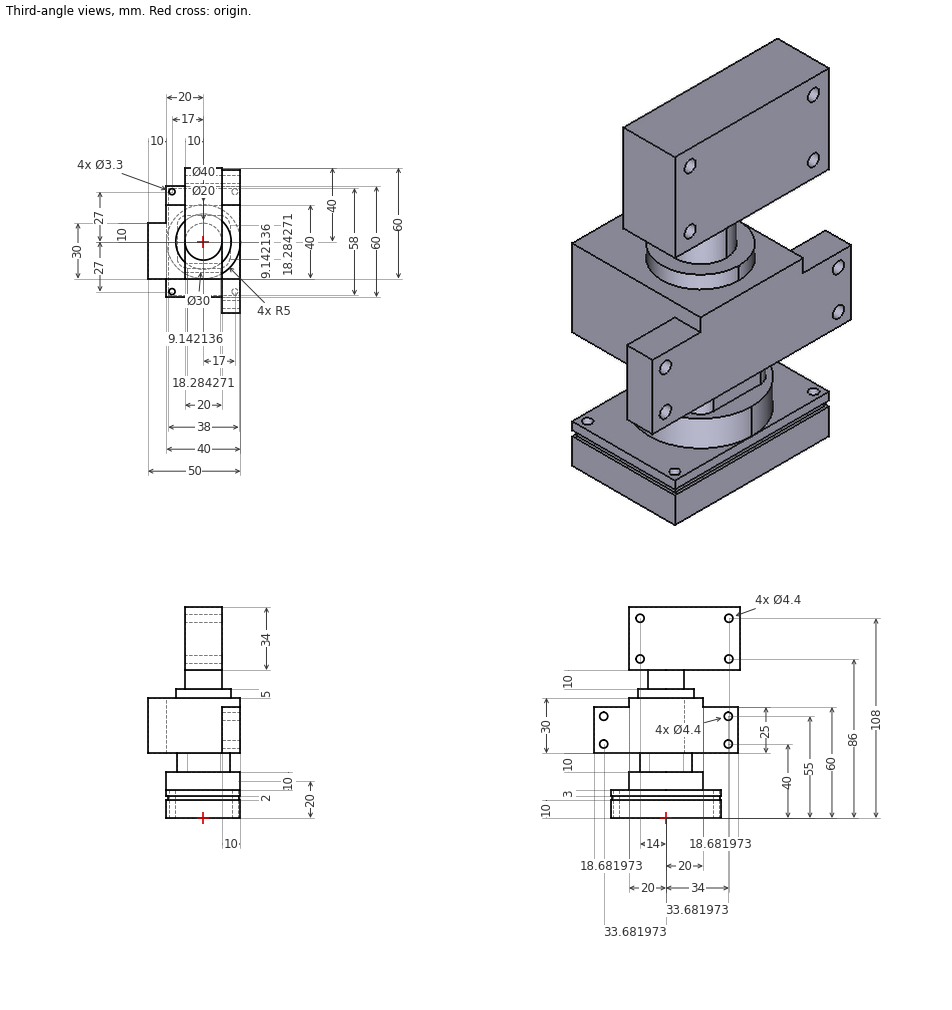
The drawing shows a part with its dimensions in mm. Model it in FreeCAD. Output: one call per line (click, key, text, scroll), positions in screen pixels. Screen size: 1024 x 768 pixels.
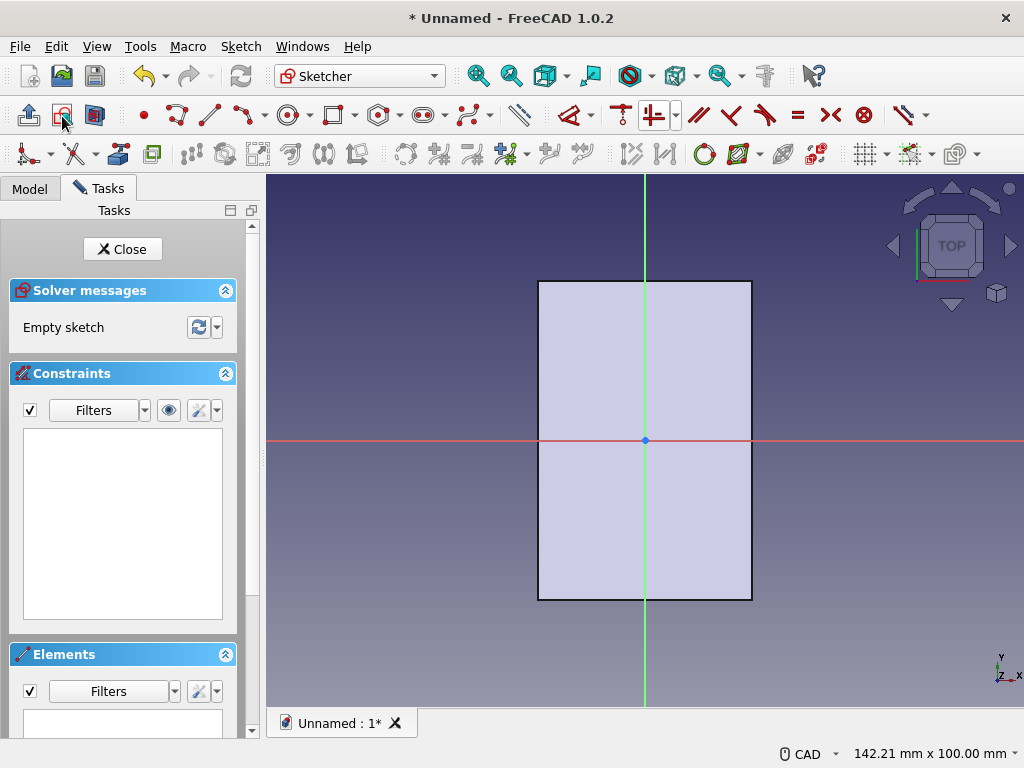
key(g)
key(v)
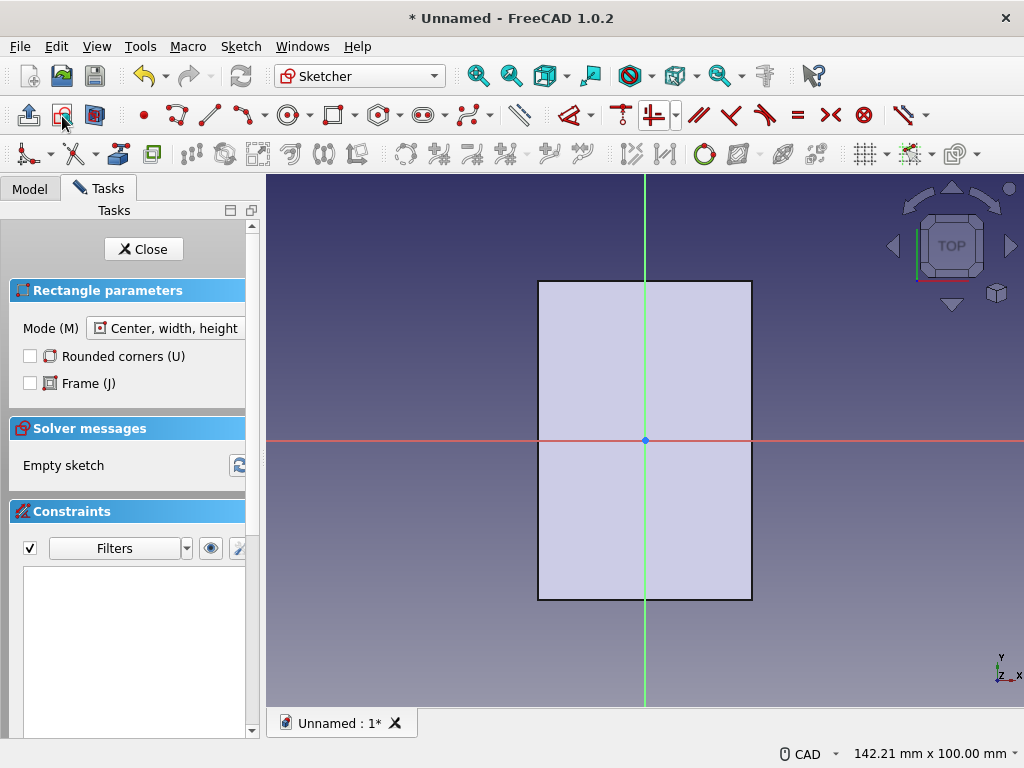
click(645, 440)
move(746, 286)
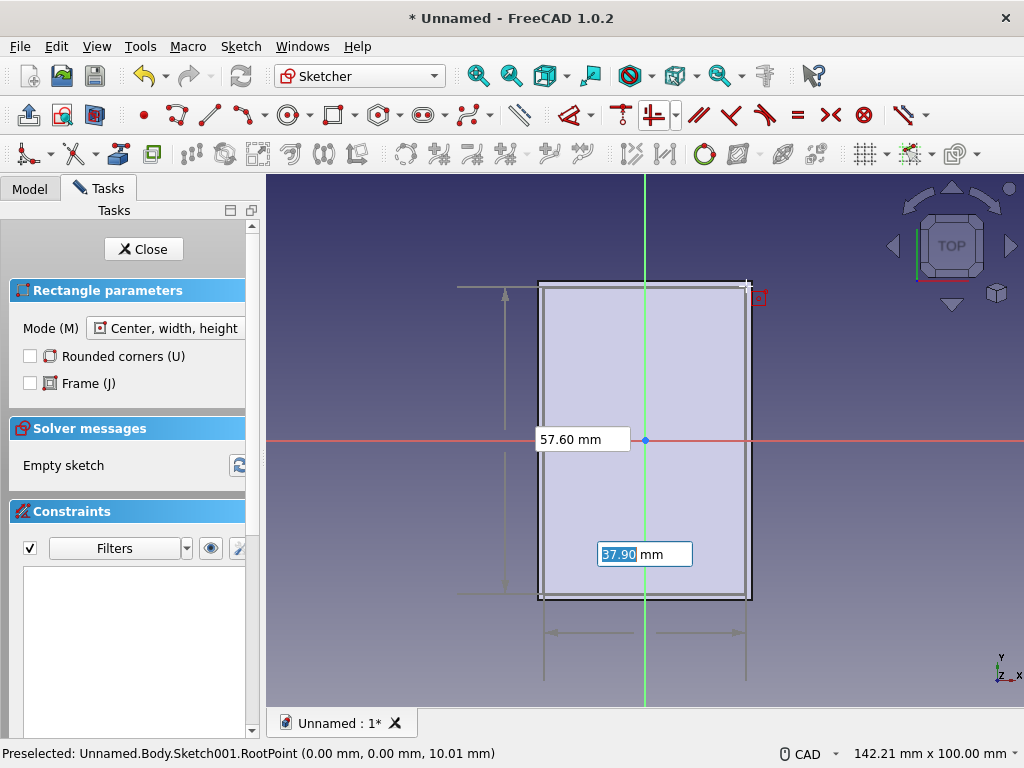
text(38)
key(Tab)
text(58)
key(Return)
key(Escape)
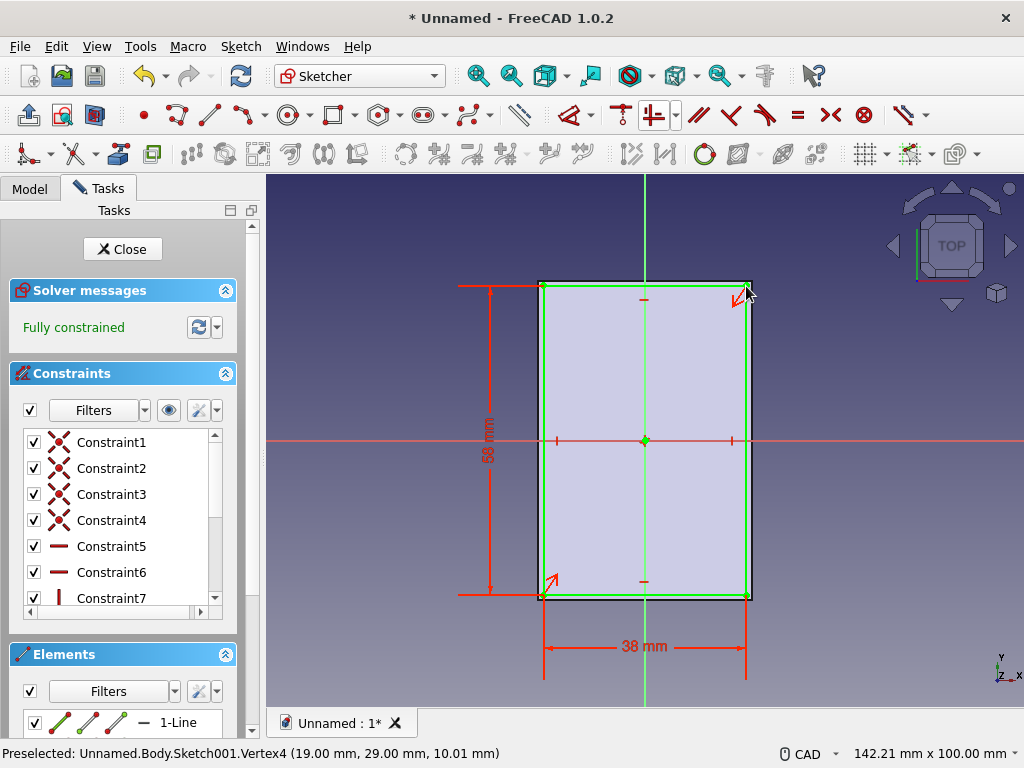
click(123, 249)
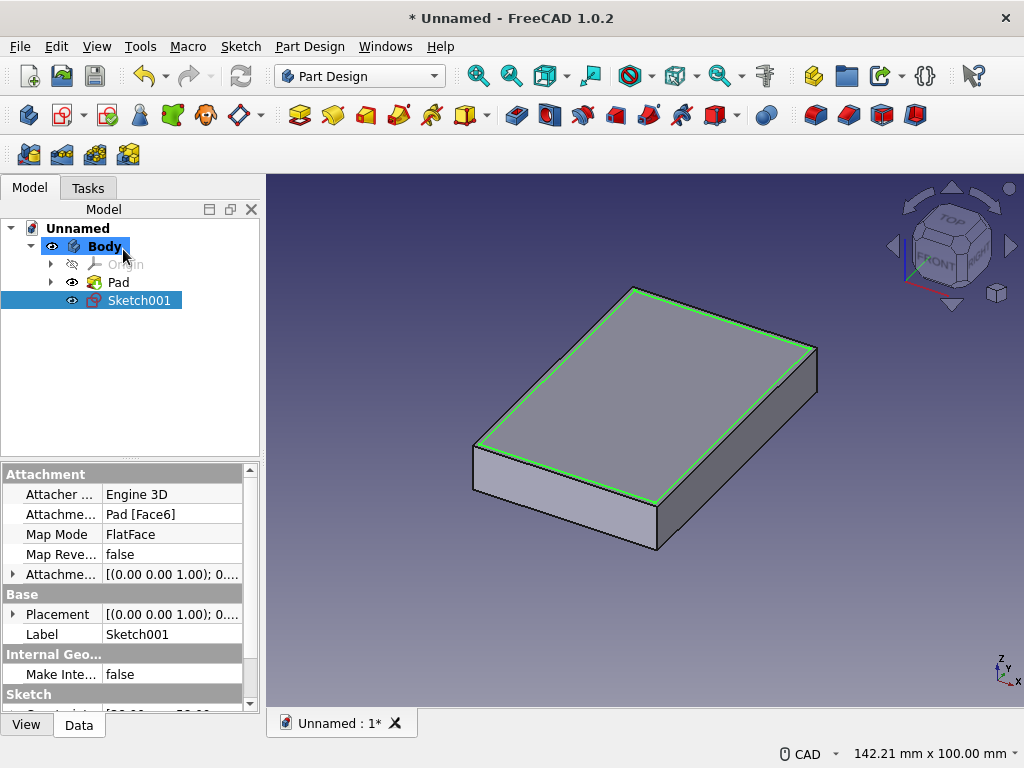
click(300, 116)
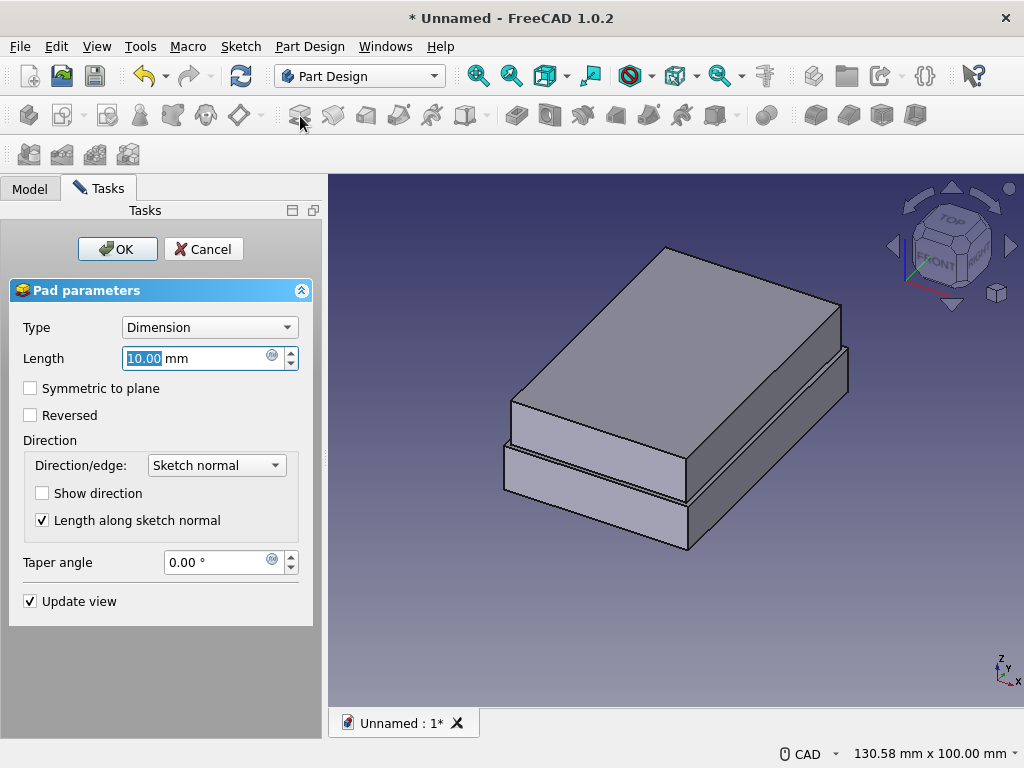
text(2)
key(Tab)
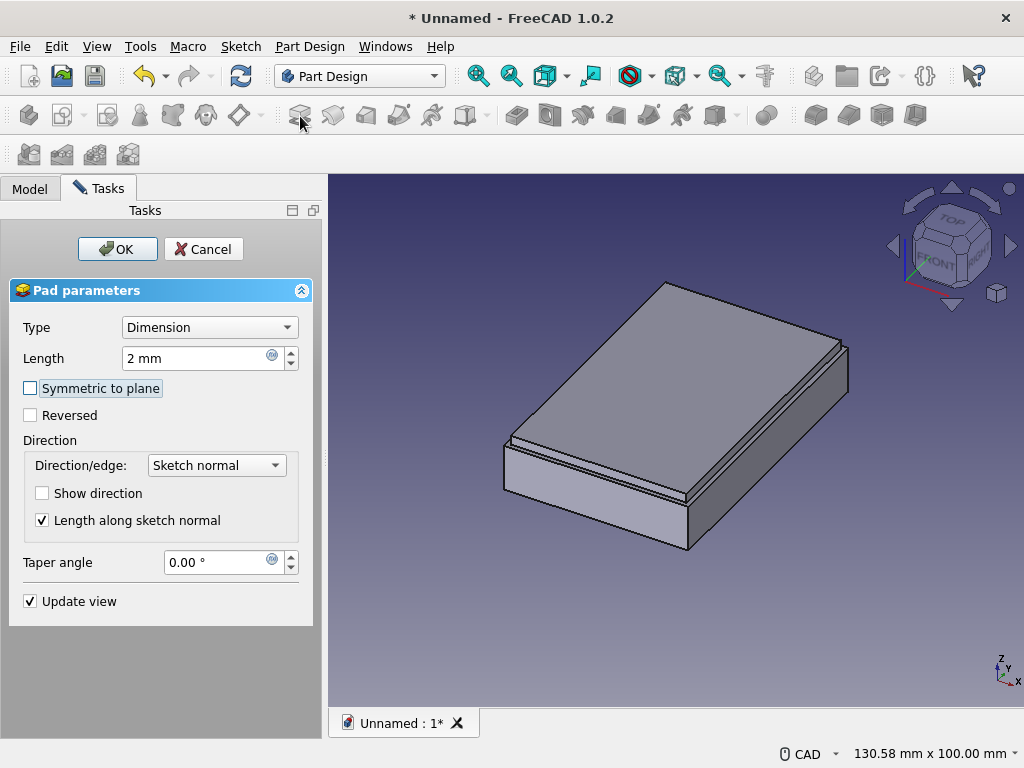
click(118, 249)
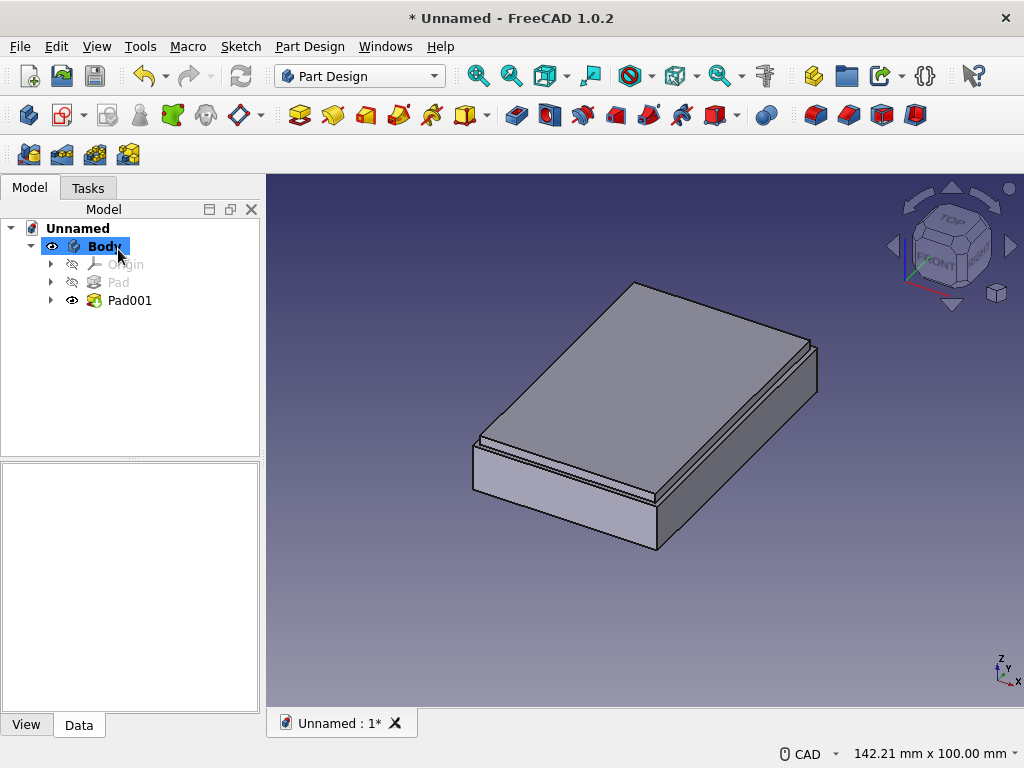
click(667, 365)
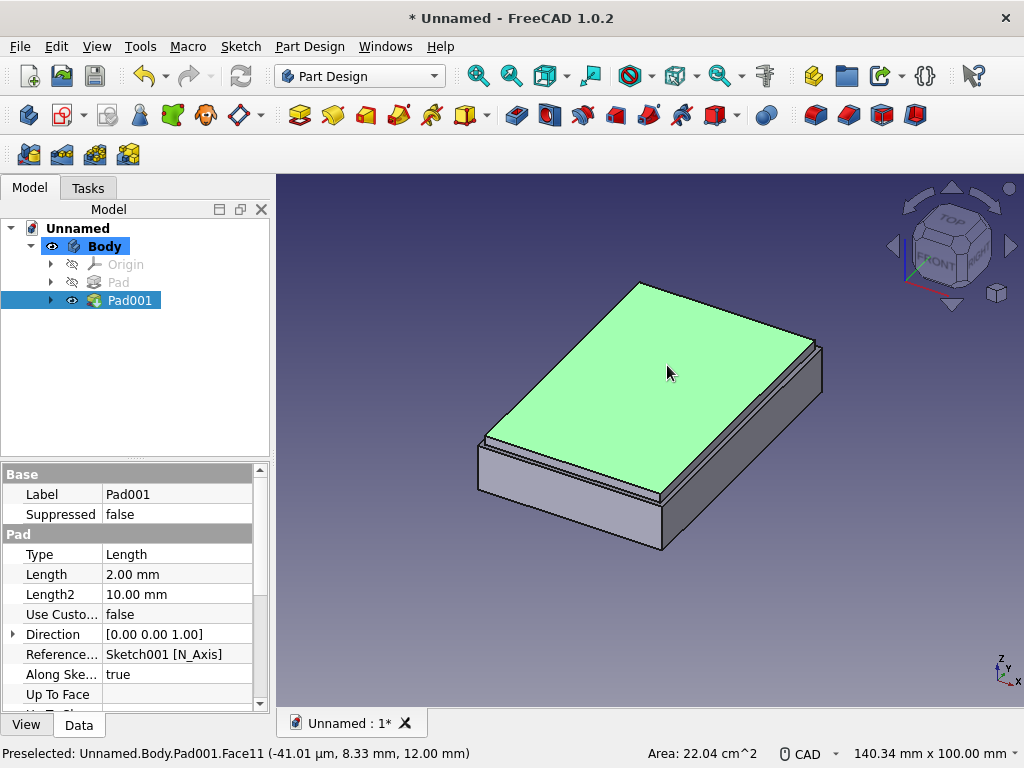
click(62, 116)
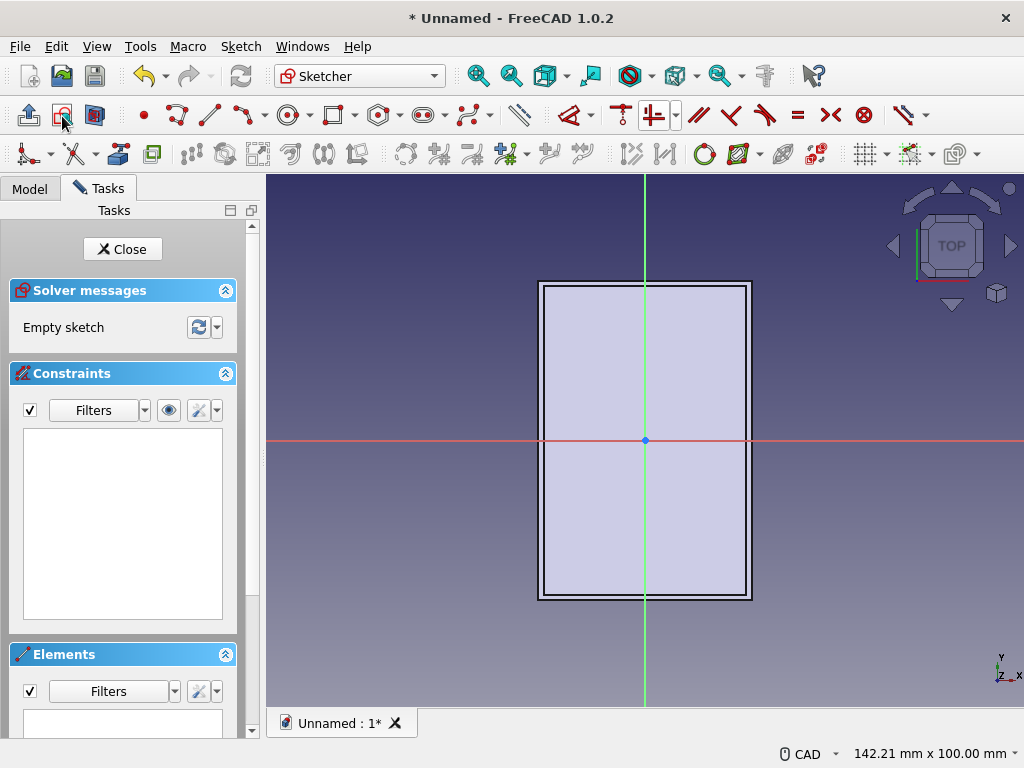
key(g)
key(v)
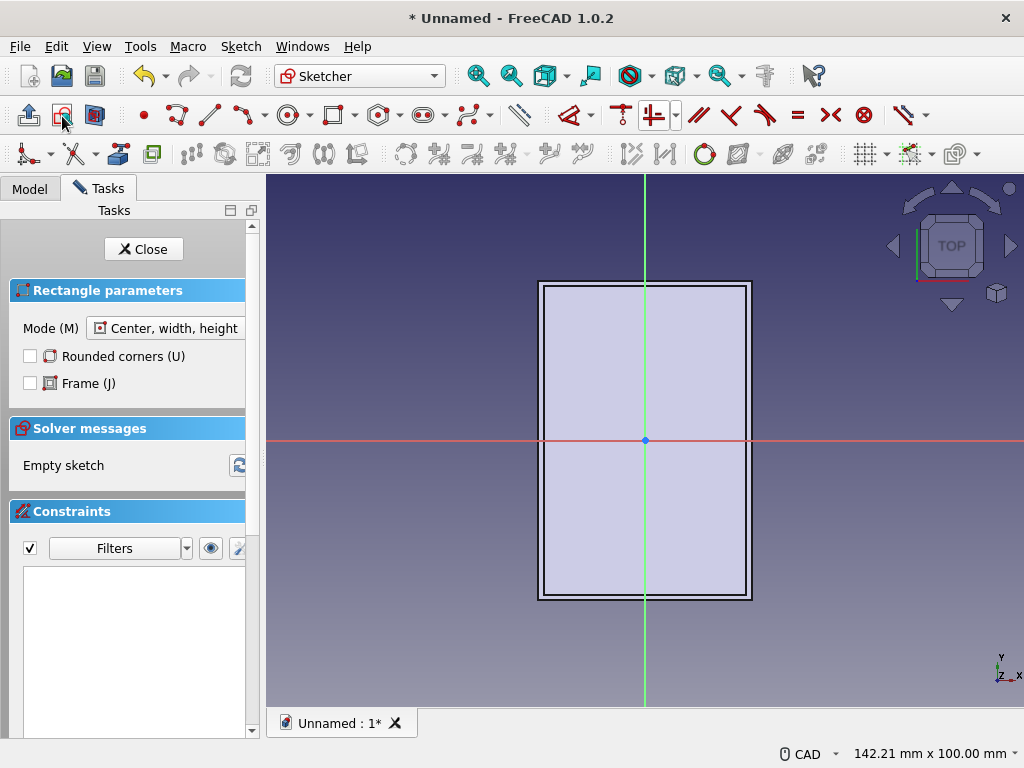
click(645, 440)
move(752, 281)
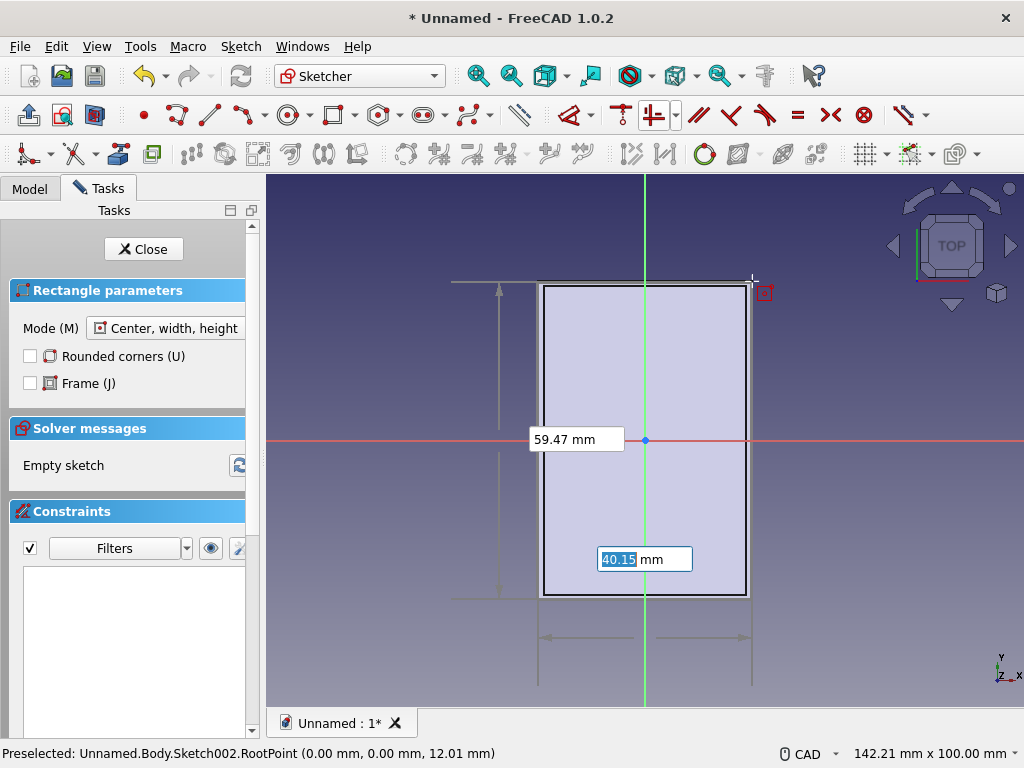
text(40)
key(Tab)
text(60)
key(Return)
key(Escape)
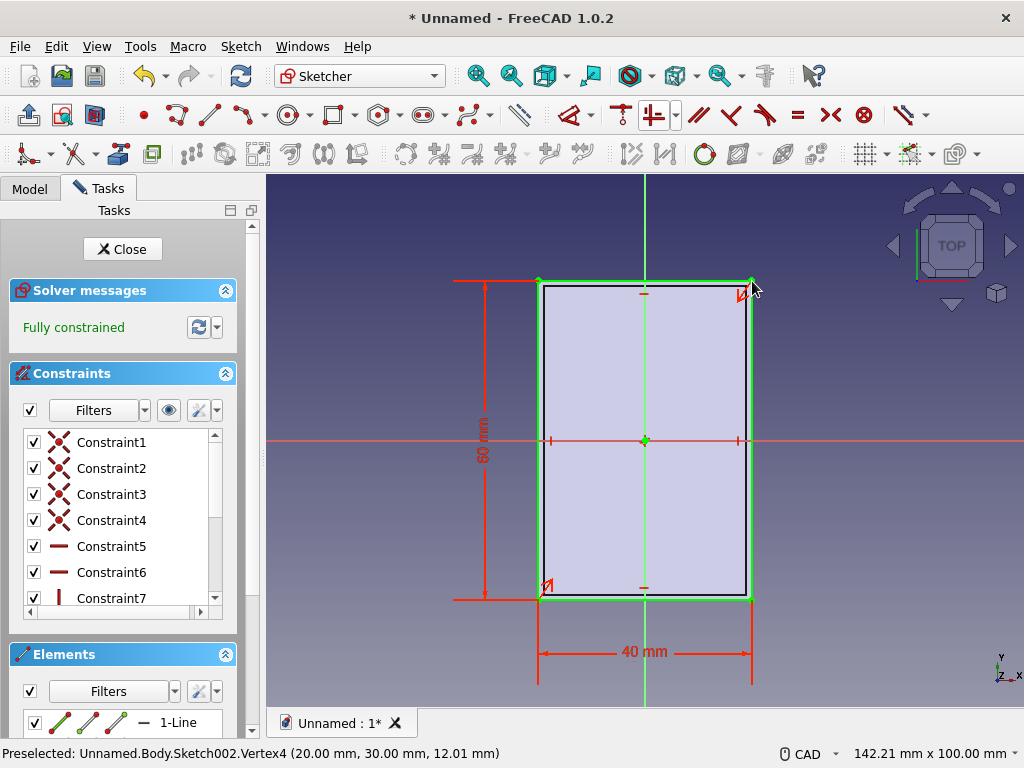
click(123, 249)